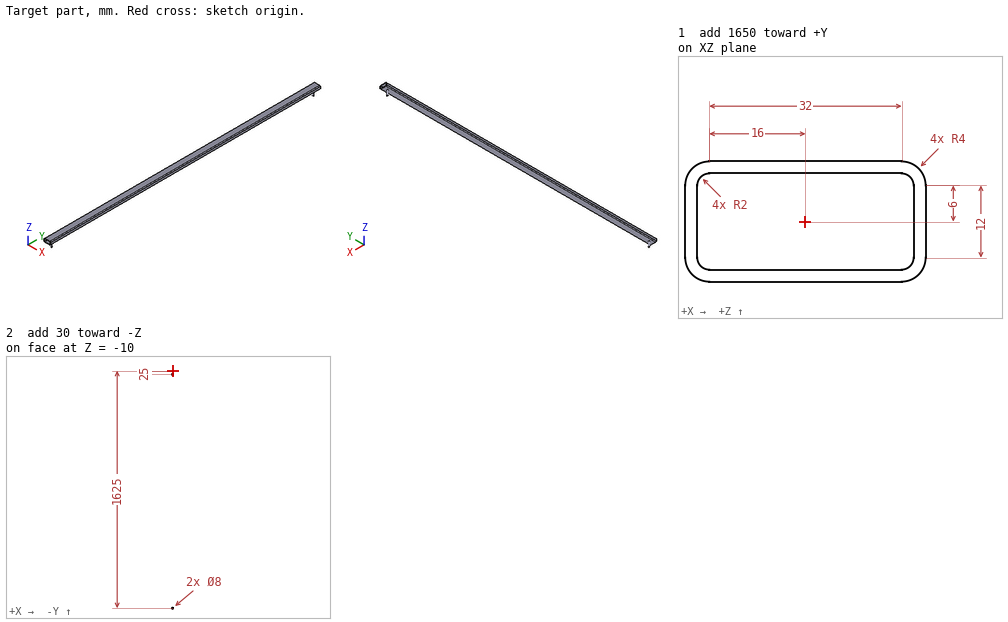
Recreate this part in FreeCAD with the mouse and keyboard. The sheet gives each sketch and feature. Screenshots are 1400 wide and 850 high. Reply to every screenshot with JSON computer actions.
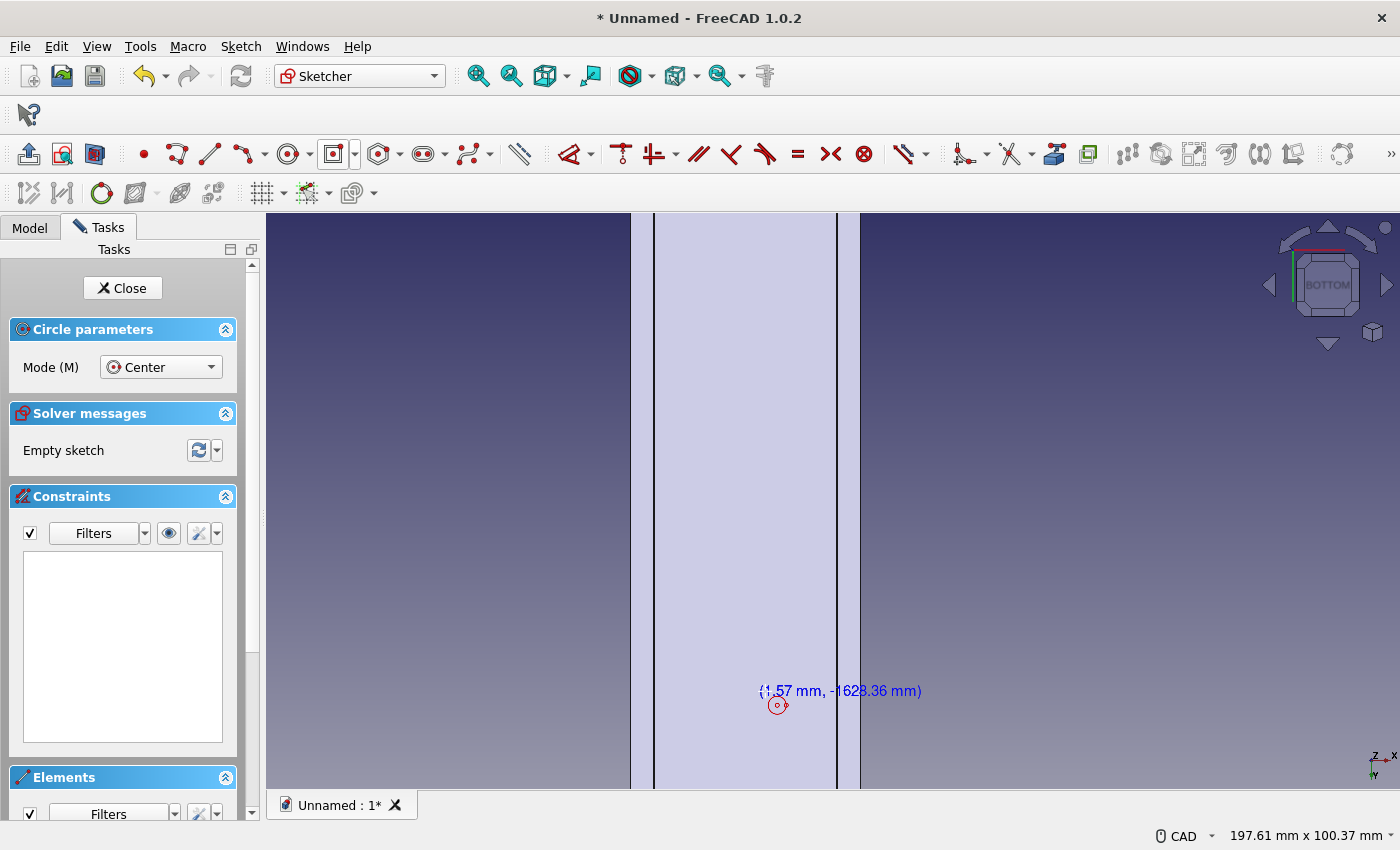
{"action": "scroll", "coordinate": [765, 735], "scroll_direction": "down", "scroll_amount": 15}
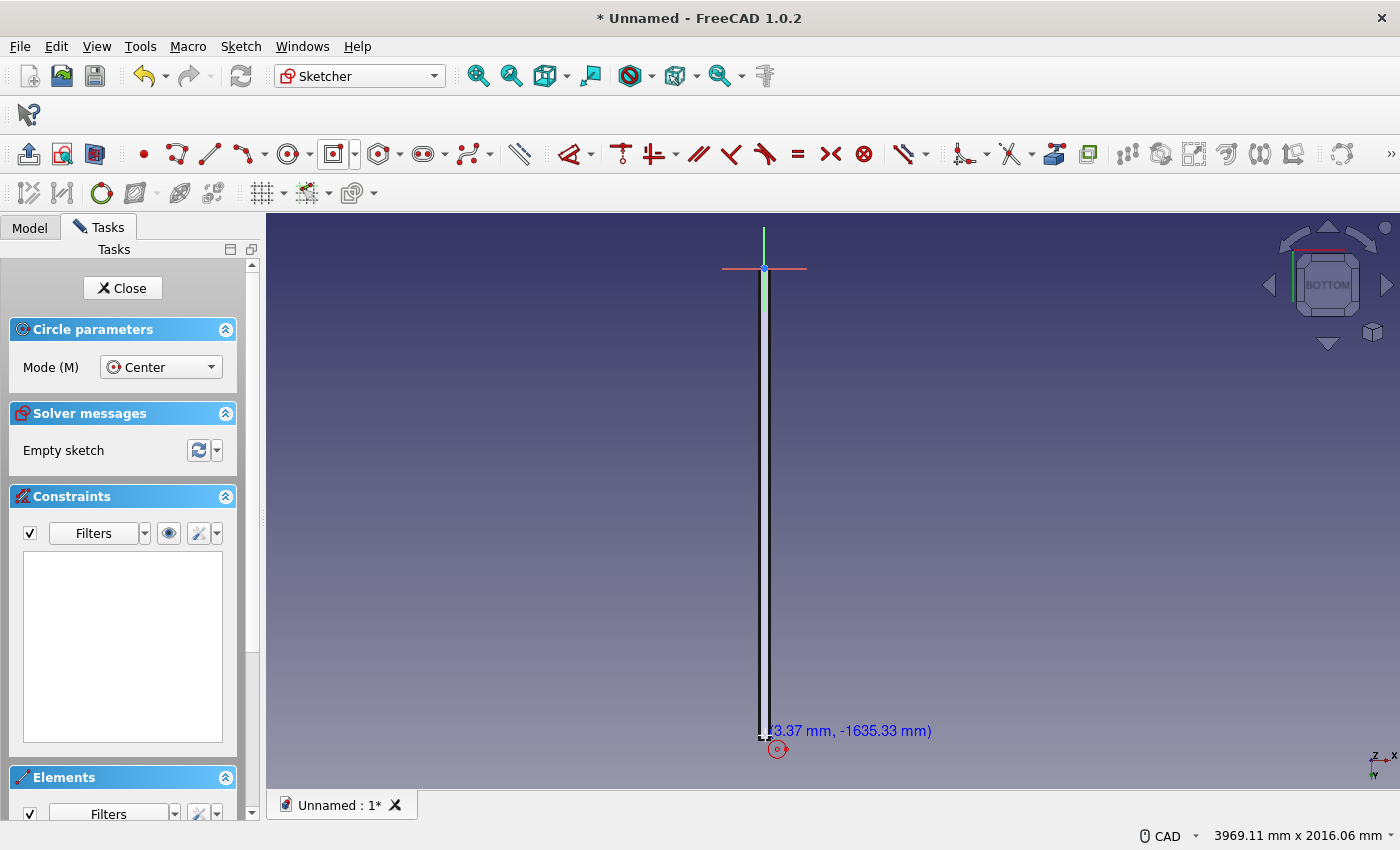
{"action": "left_click", "coordinate": [764, 733]}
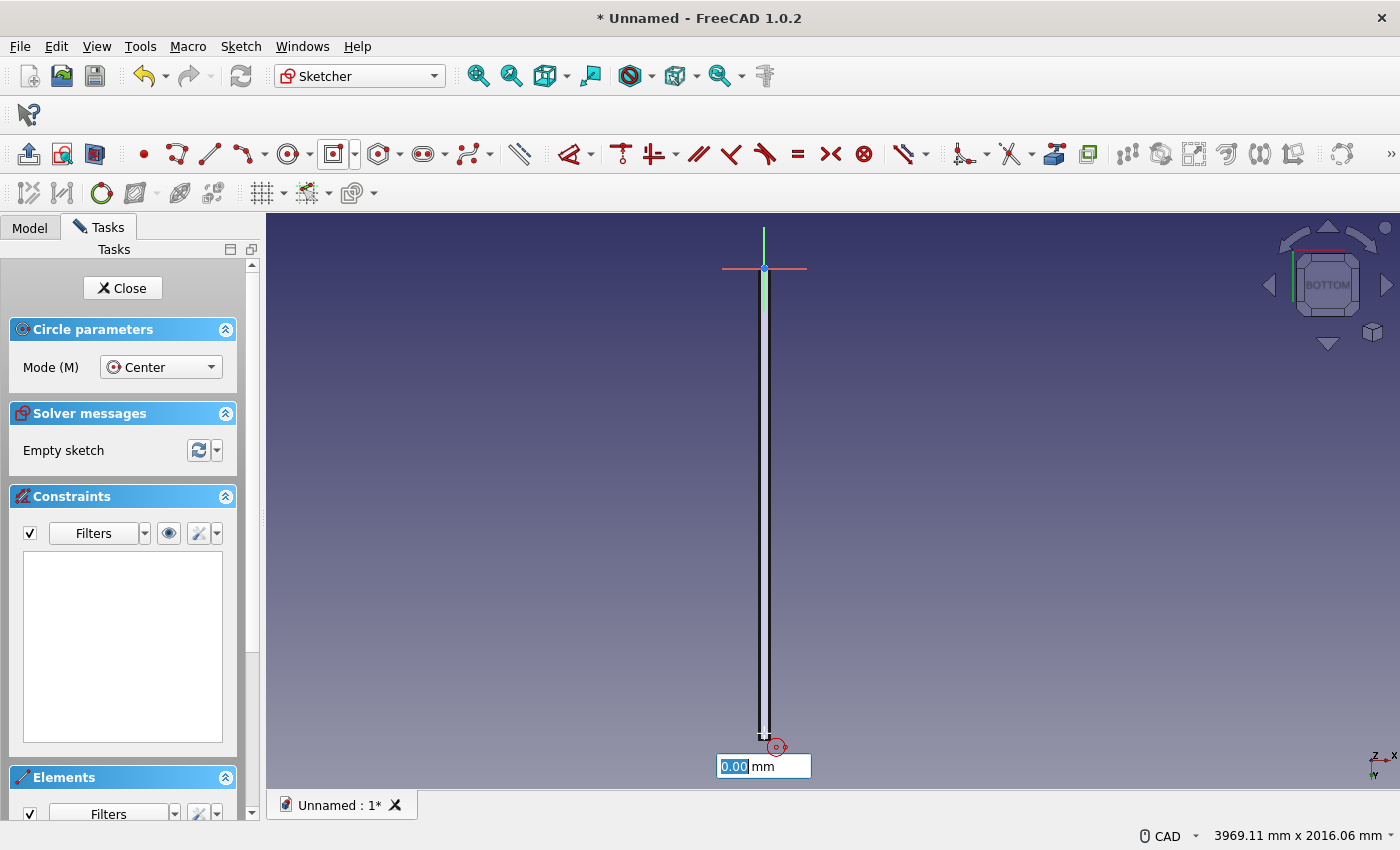
{"action": "scroll", "coordinate": [766, 733], "scroll_direction": "up", "scroll_amount": 14}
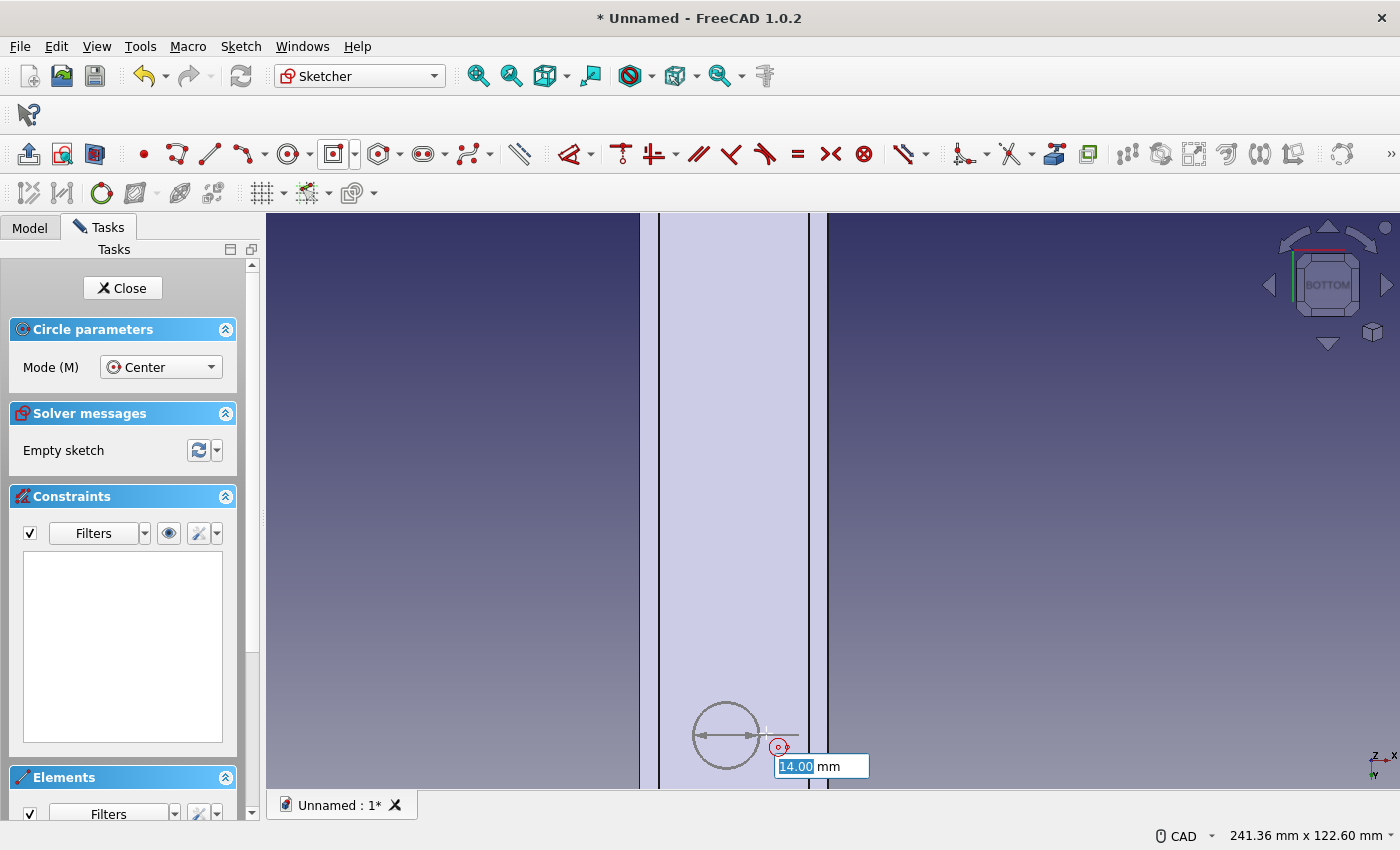
{"action": "left_click", "coordinate": [751, 712]}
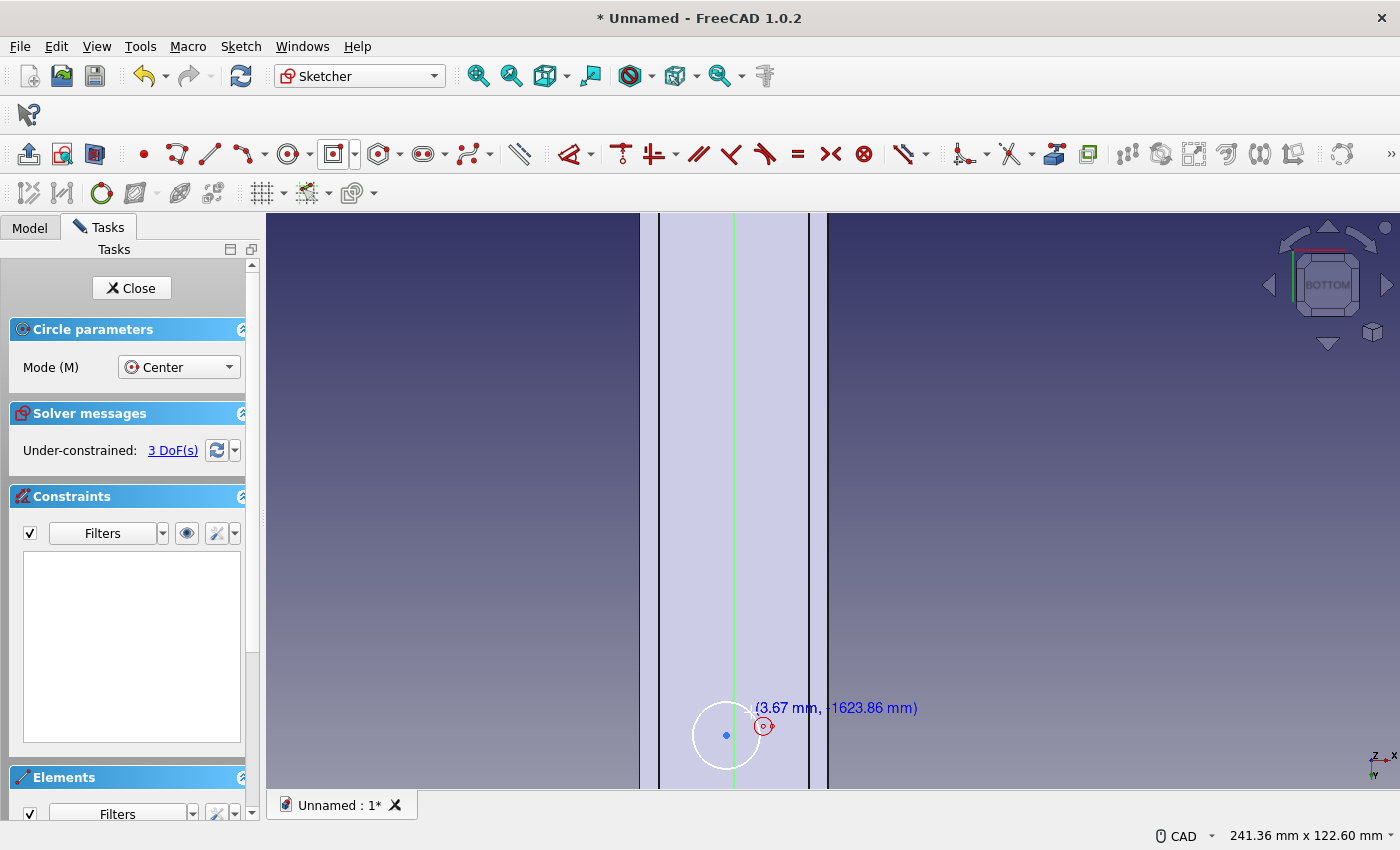
{"action": "scroll", "coordinate": [766, 689], "scroll_direction": "down", "scroll_amount": 15}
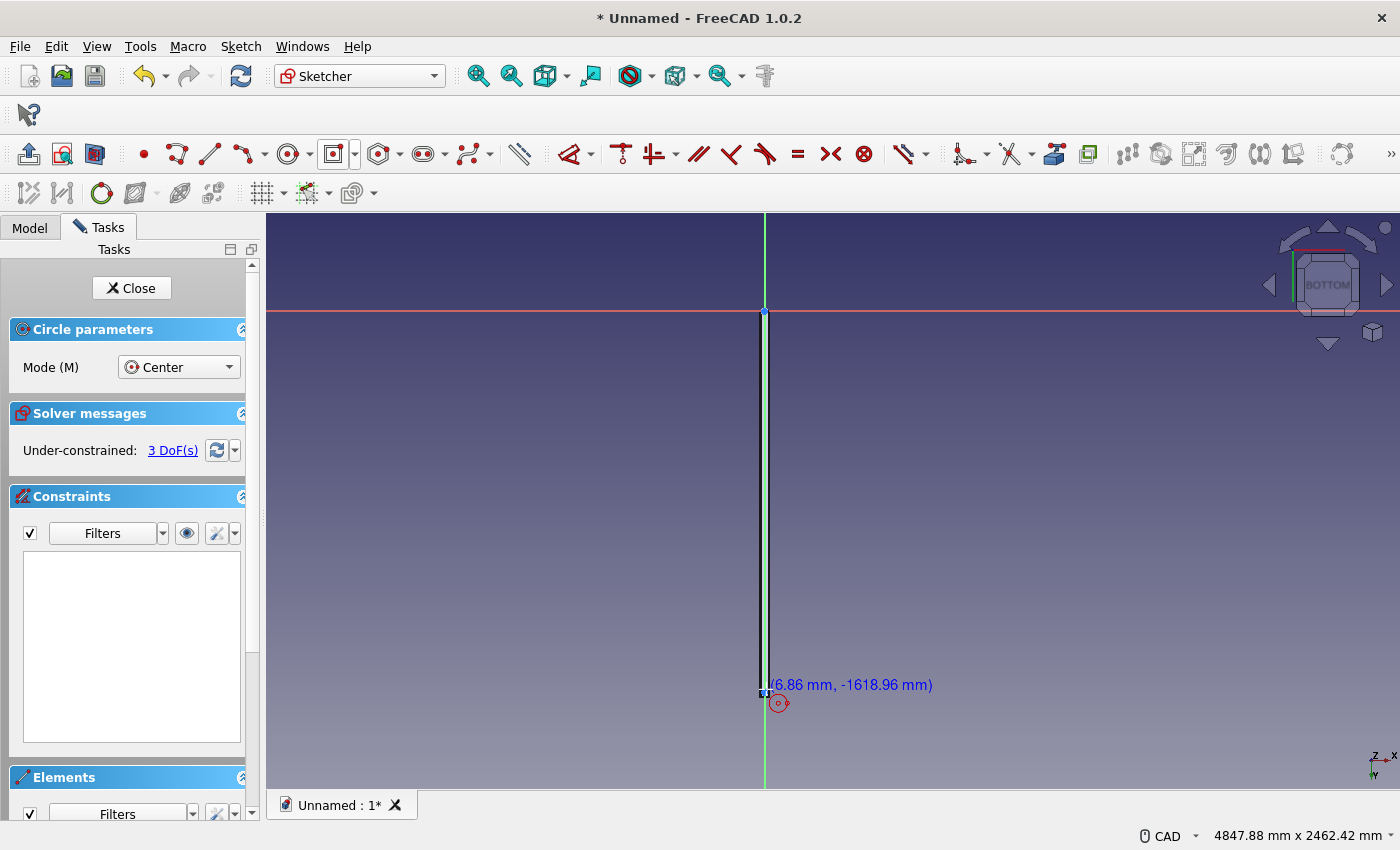
{"action": "scroll", "coordinate": [765, 317], "scroll_direction": "up", "scroll_amount": 16}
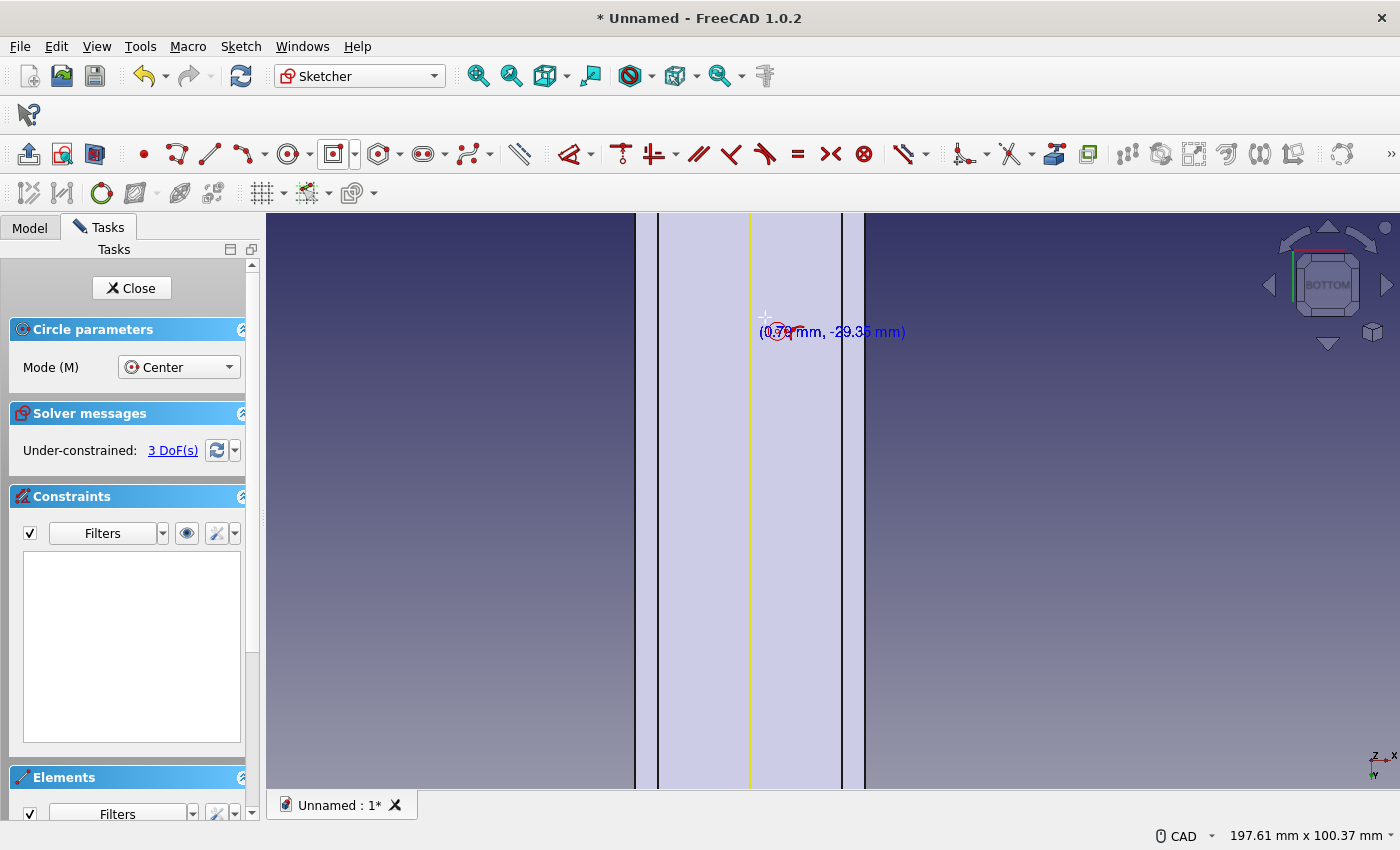
{"action": "scroll", "coordinate": [765, 274], "scroll_direction": "down", "scroll_amount": 15}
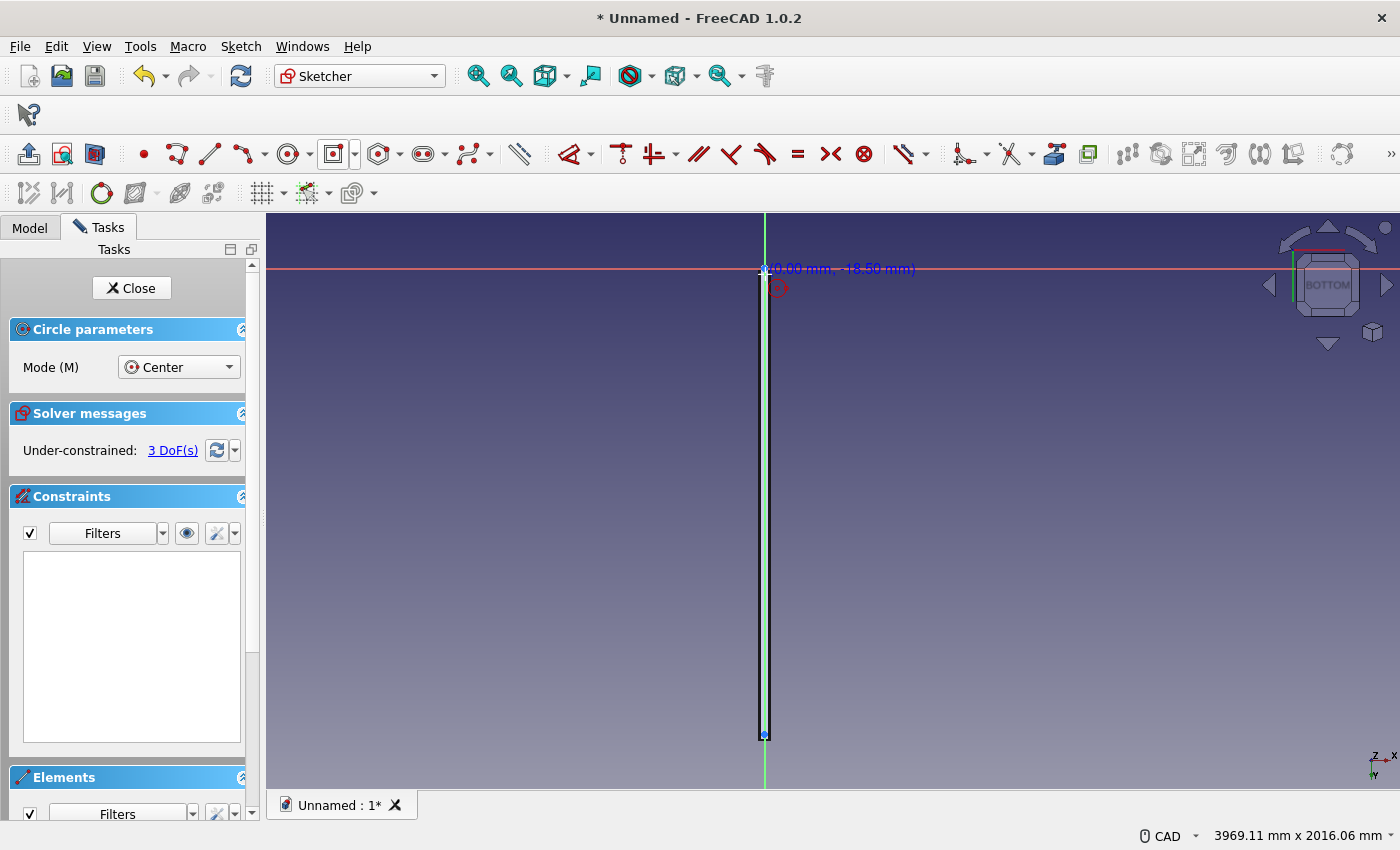
{"action": "scroll", "coordinate": [765, 276], "scroll_direction": "up", "scroll_amount": 4}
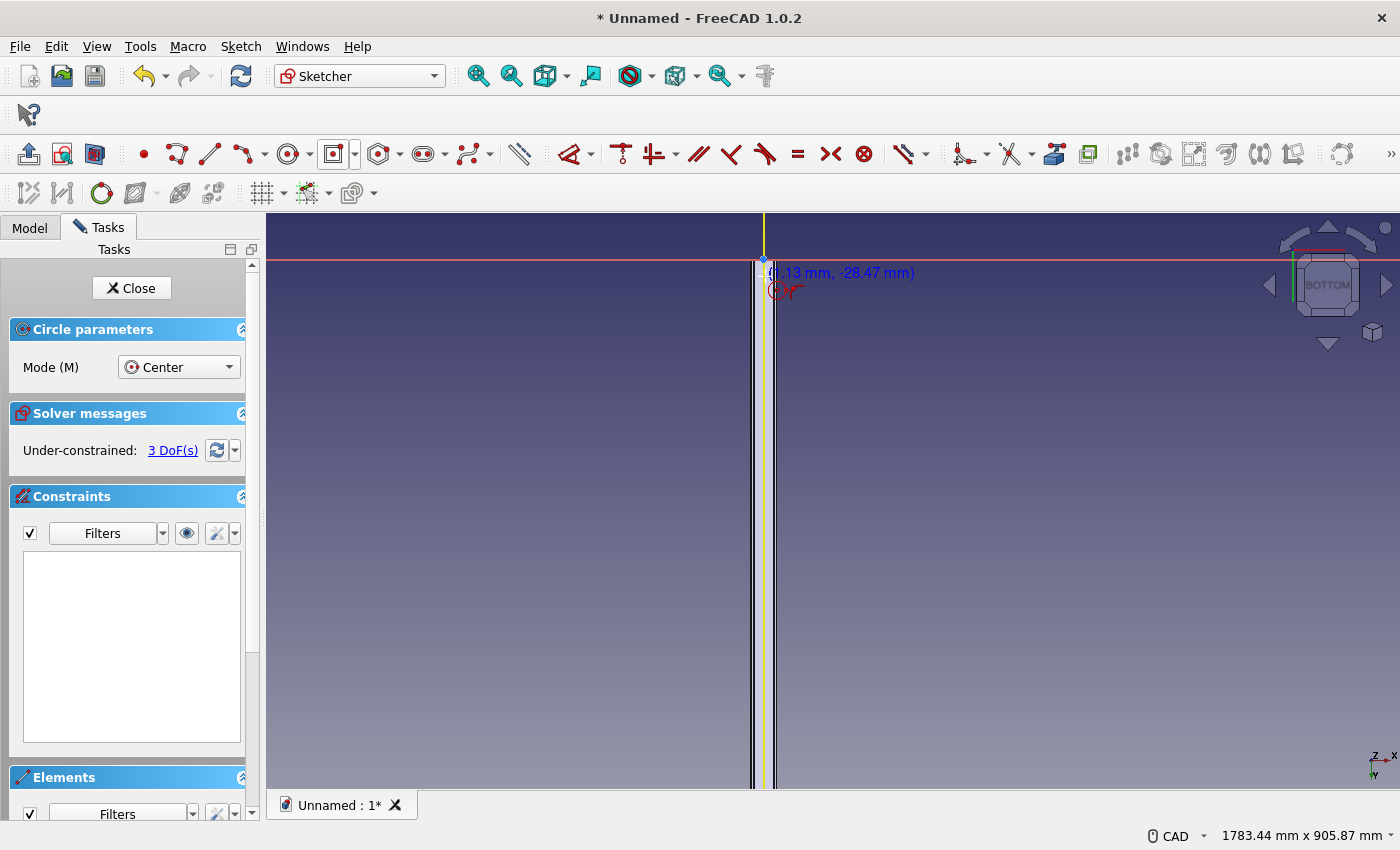
{"action": "left_click", "coordinate": [764, 276]}